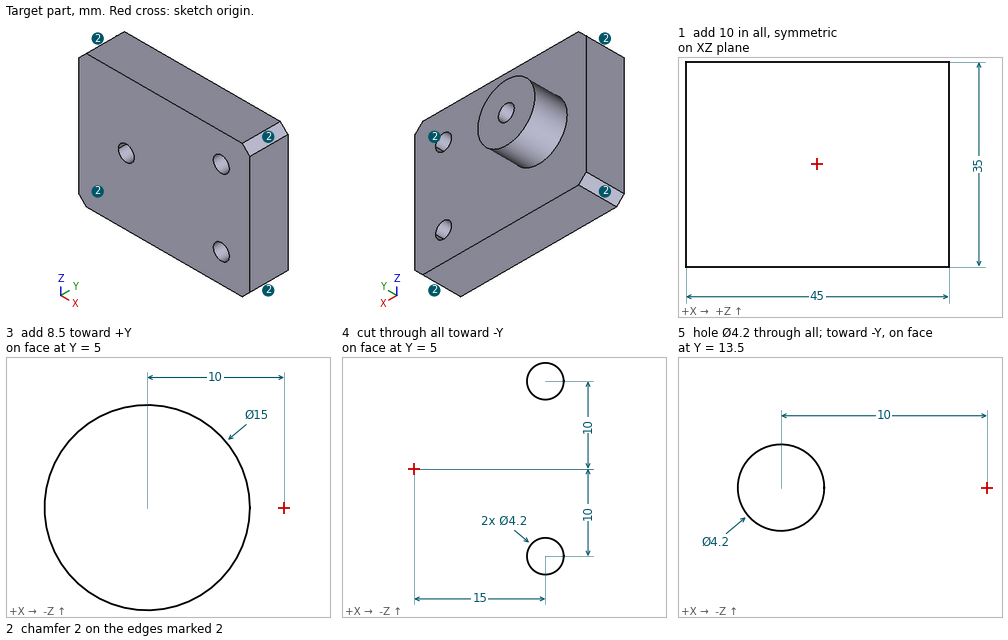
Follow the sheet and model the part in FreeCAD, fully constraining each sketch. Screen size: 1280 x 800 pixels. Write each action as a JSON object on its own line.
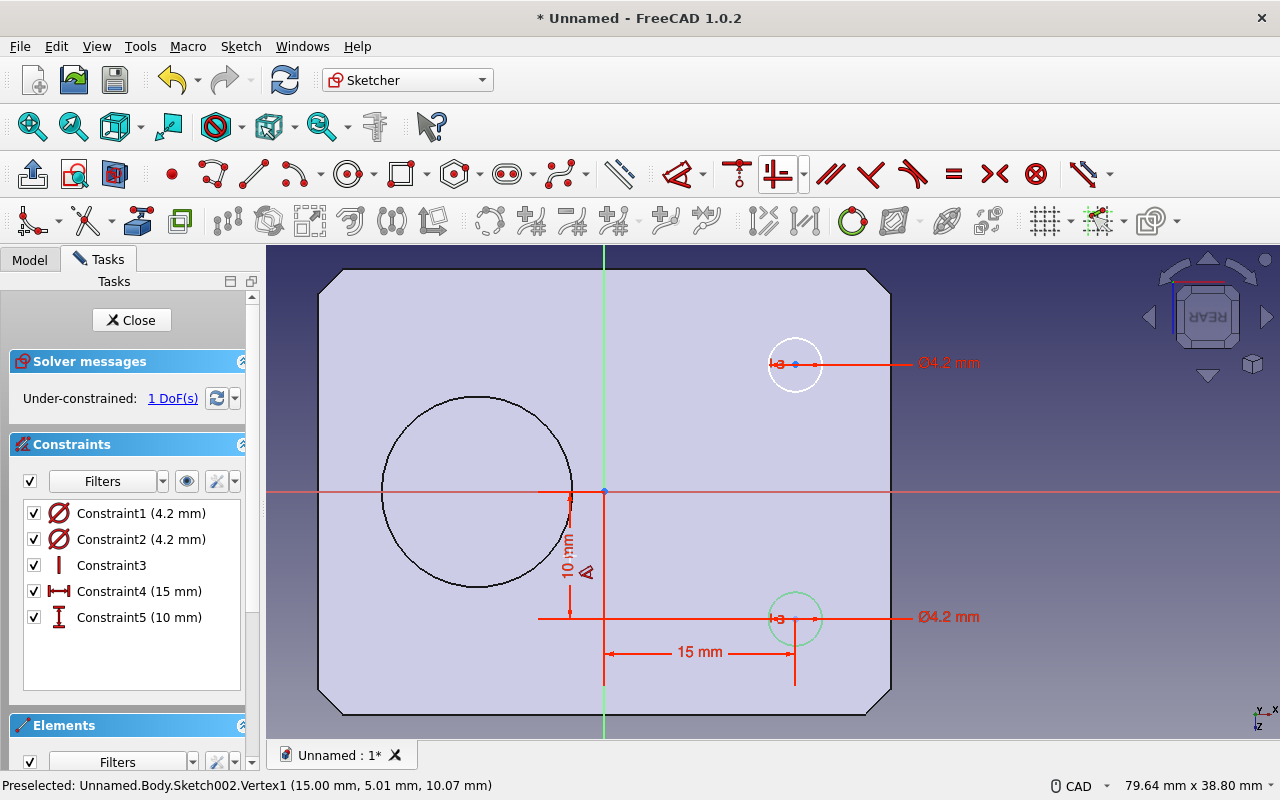
{"action": "left_click", "coordinate": [795, 365]}
{"action": "left_click", "coordinate": [570, 428]}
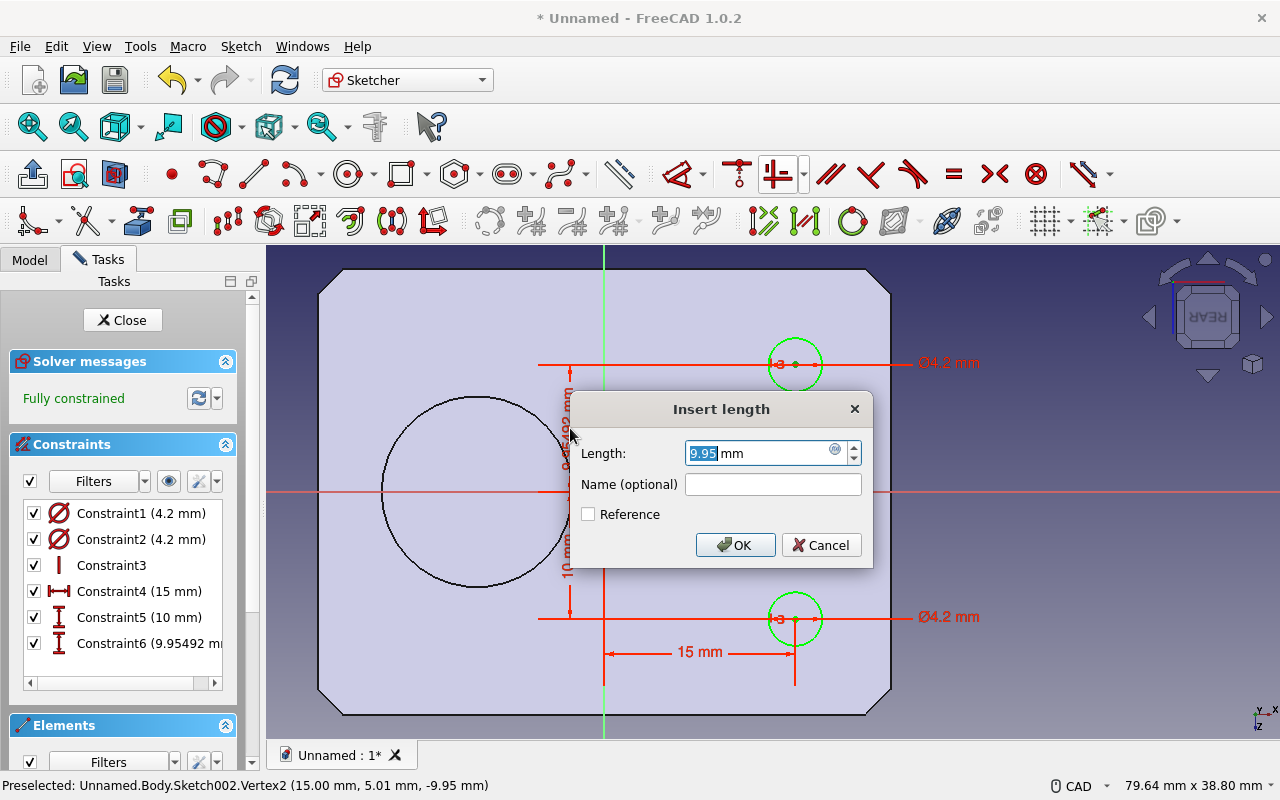
{"action": "type", "text": "10"}
{"action": "key", "text": "Return"}
{"action": "key", "text": "Escape"}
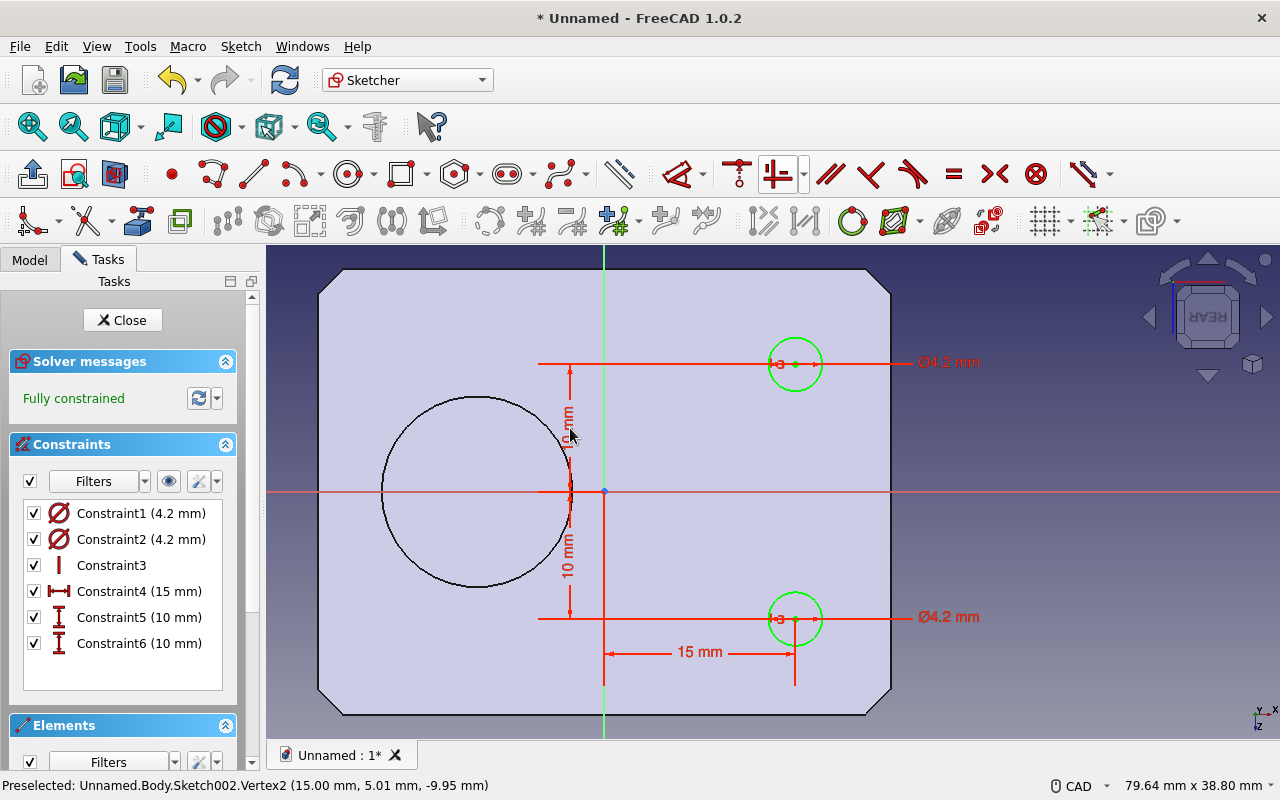
{"action": "left_click", "coordinate": [123, 320]}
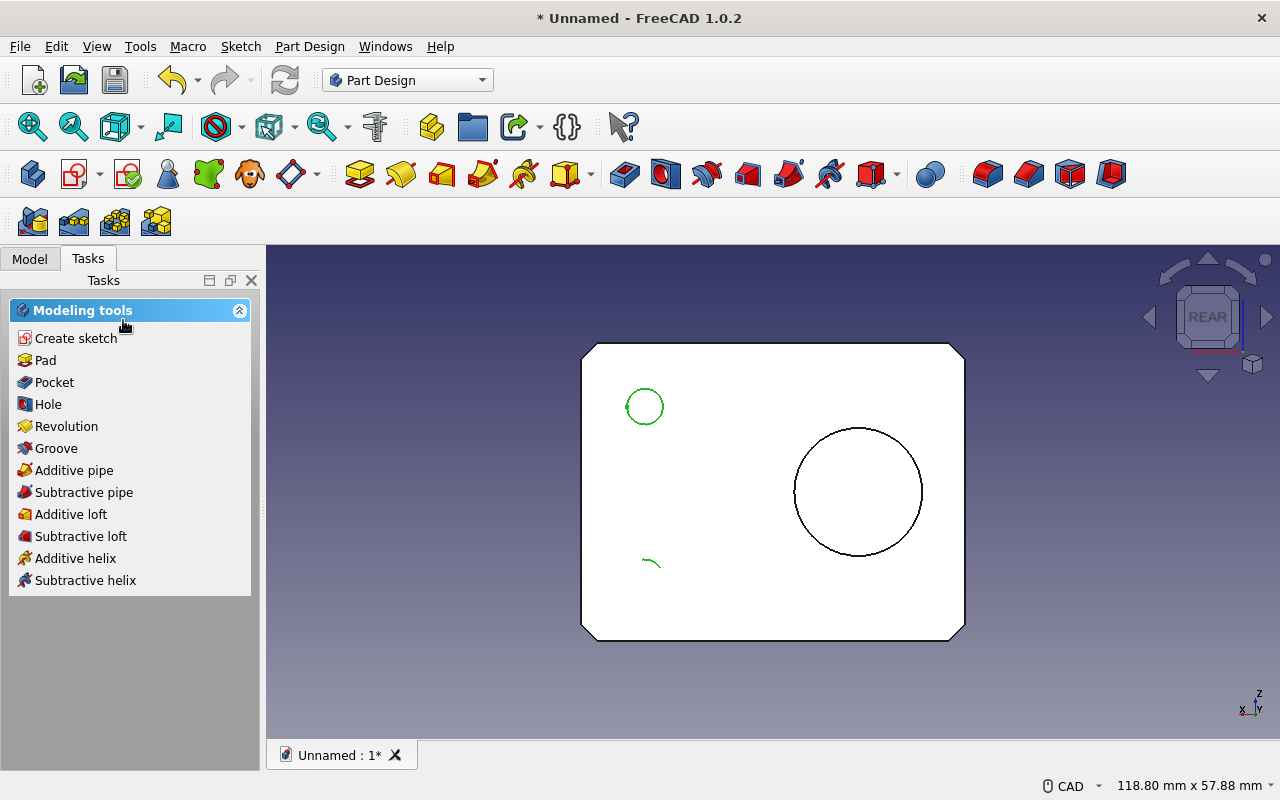
{"action": "left_click", "coordinate": [625, 174]}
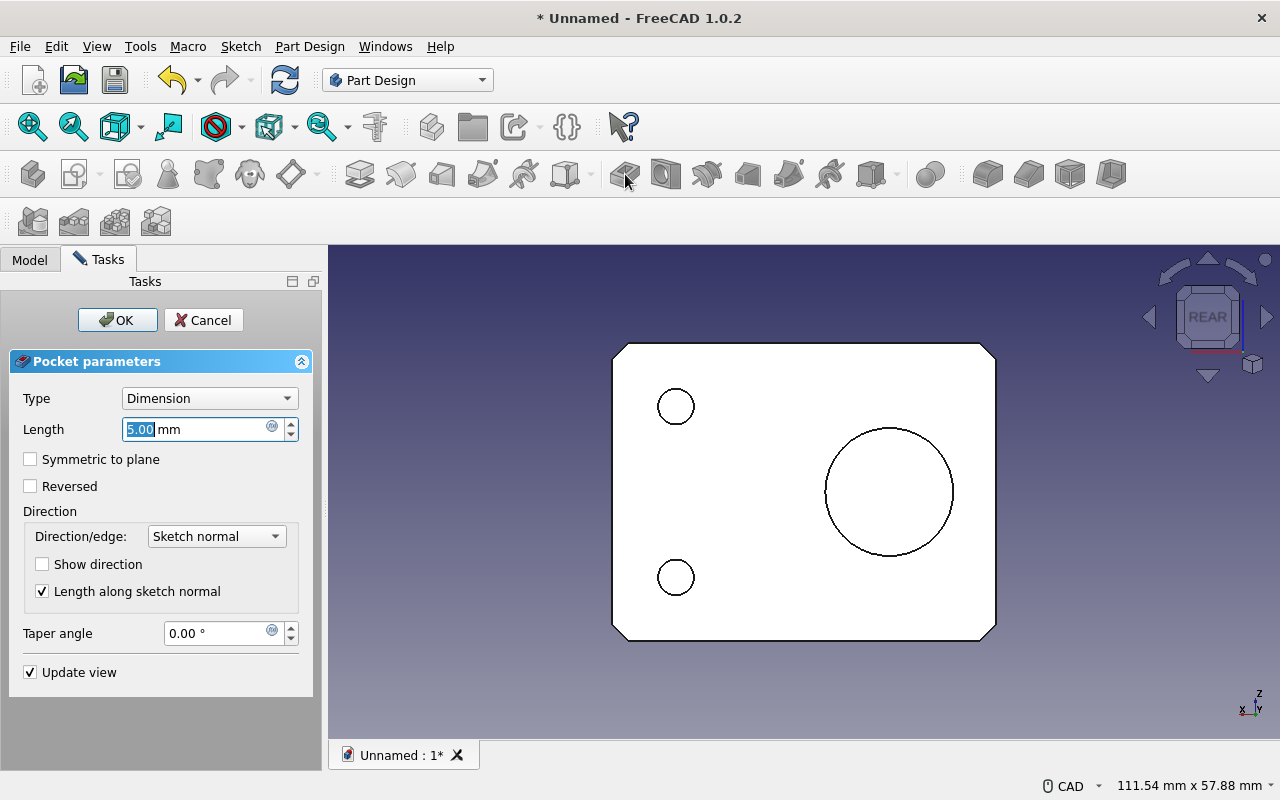
{"action": "left_click", "coordinate": [210, 398]}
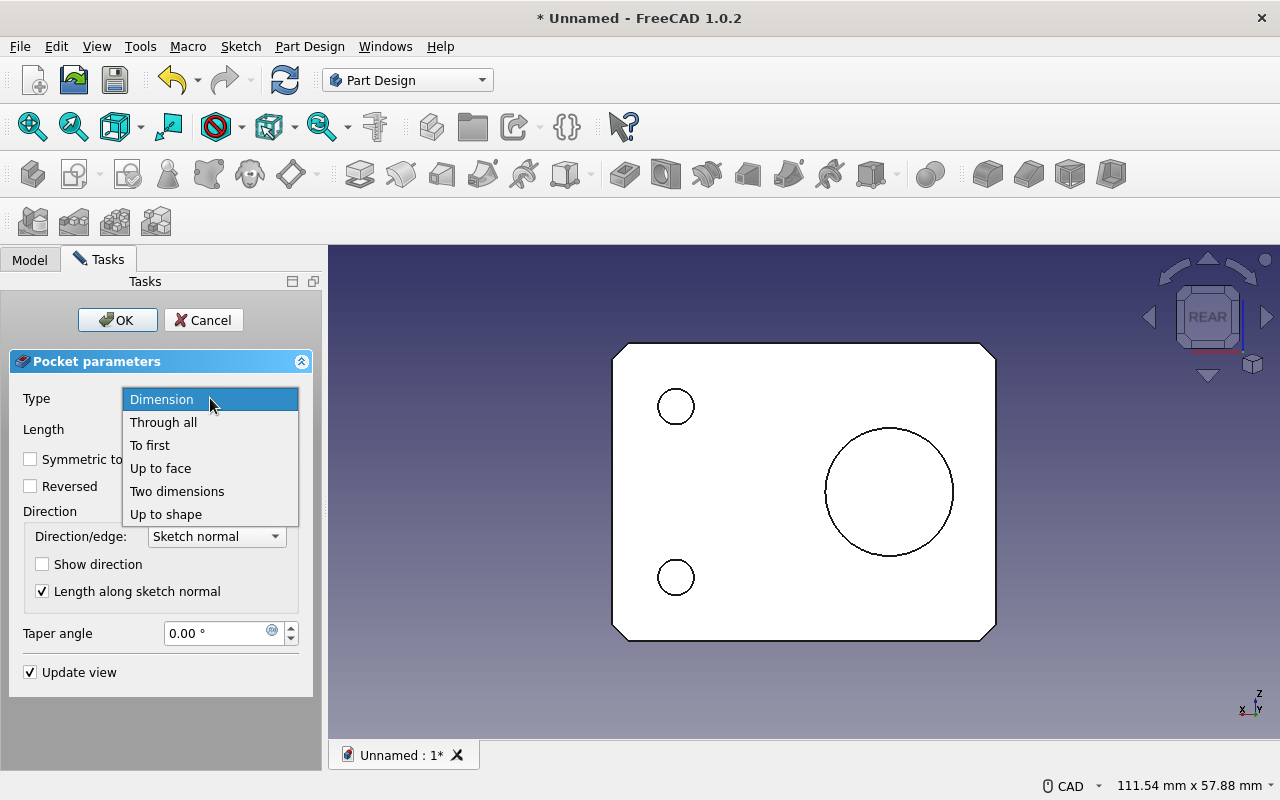
{"action": "left_click", "coordinate": [208, 422]}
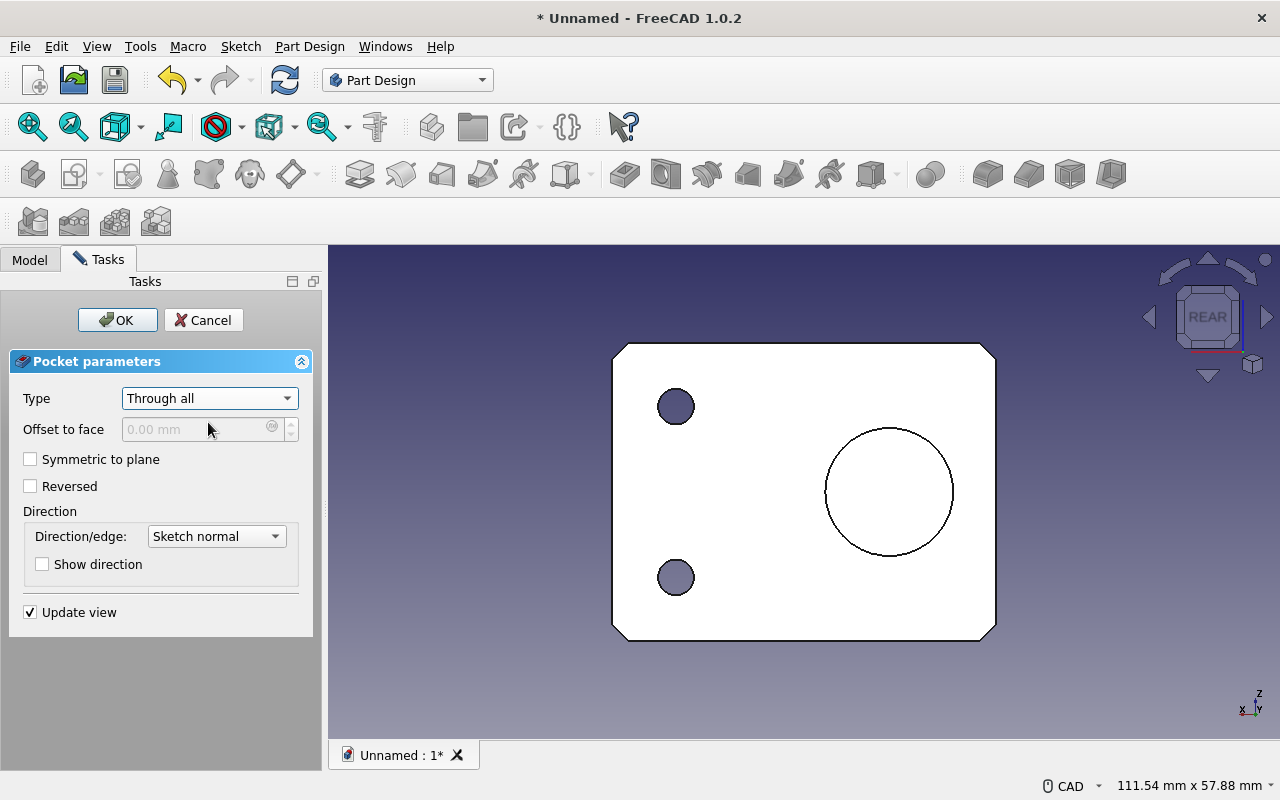
{"action": "left_click", "coordinate": [118, 320]}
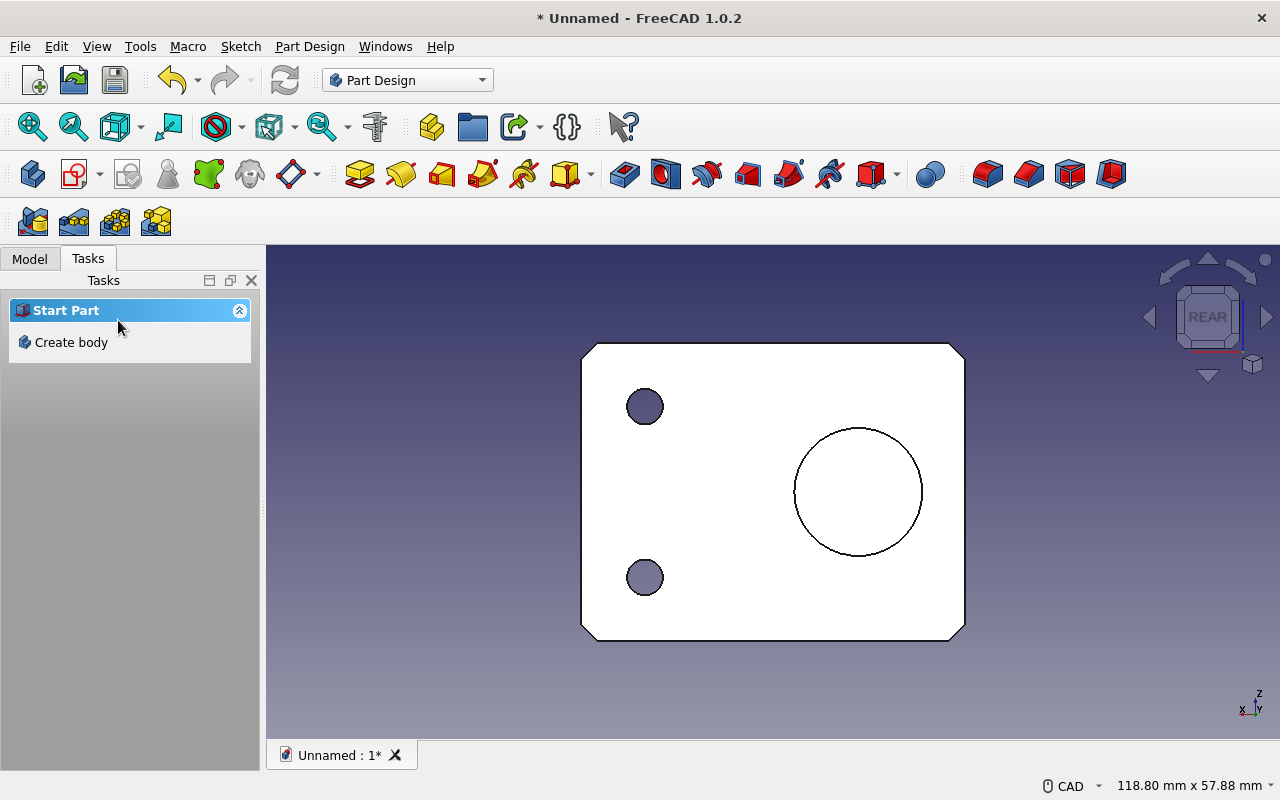
{"action": "left_click", "coordinate": [858, 491]}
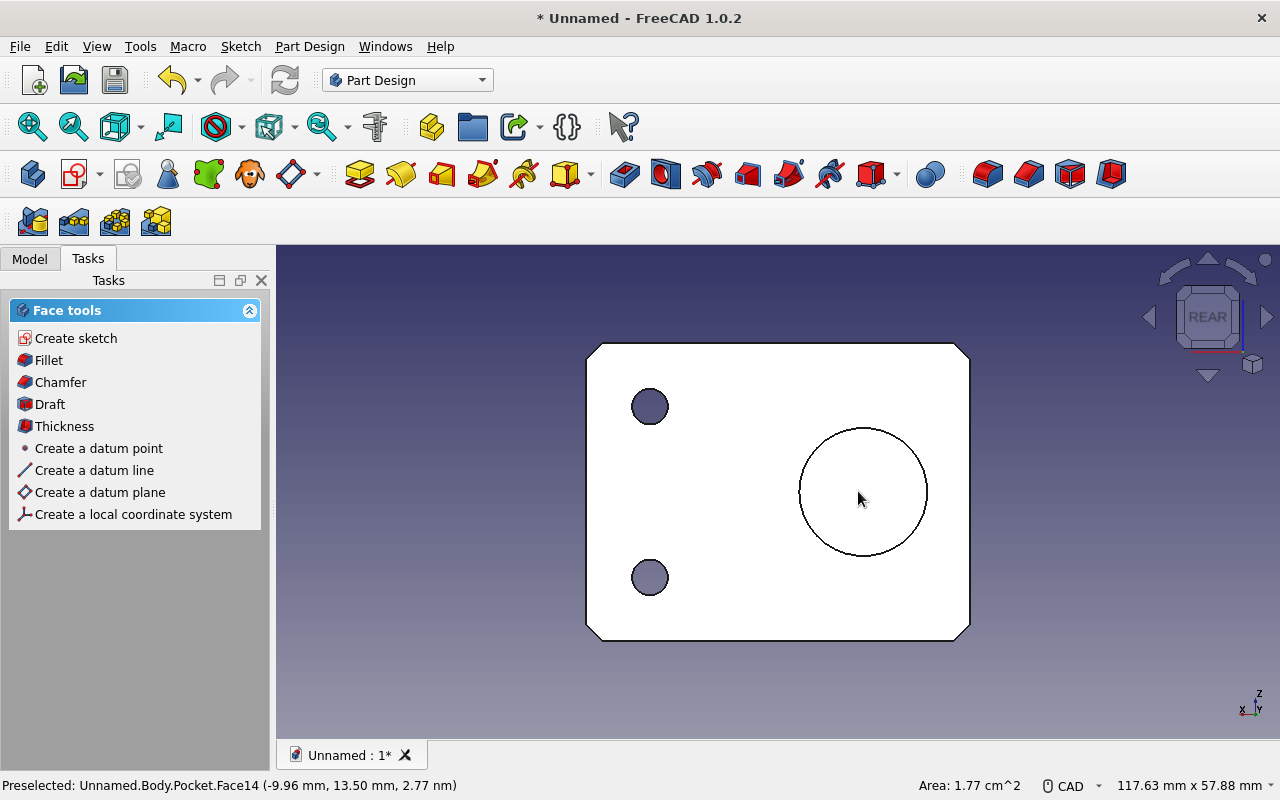
{"action": "left_click", "coordinate": [74, 174]}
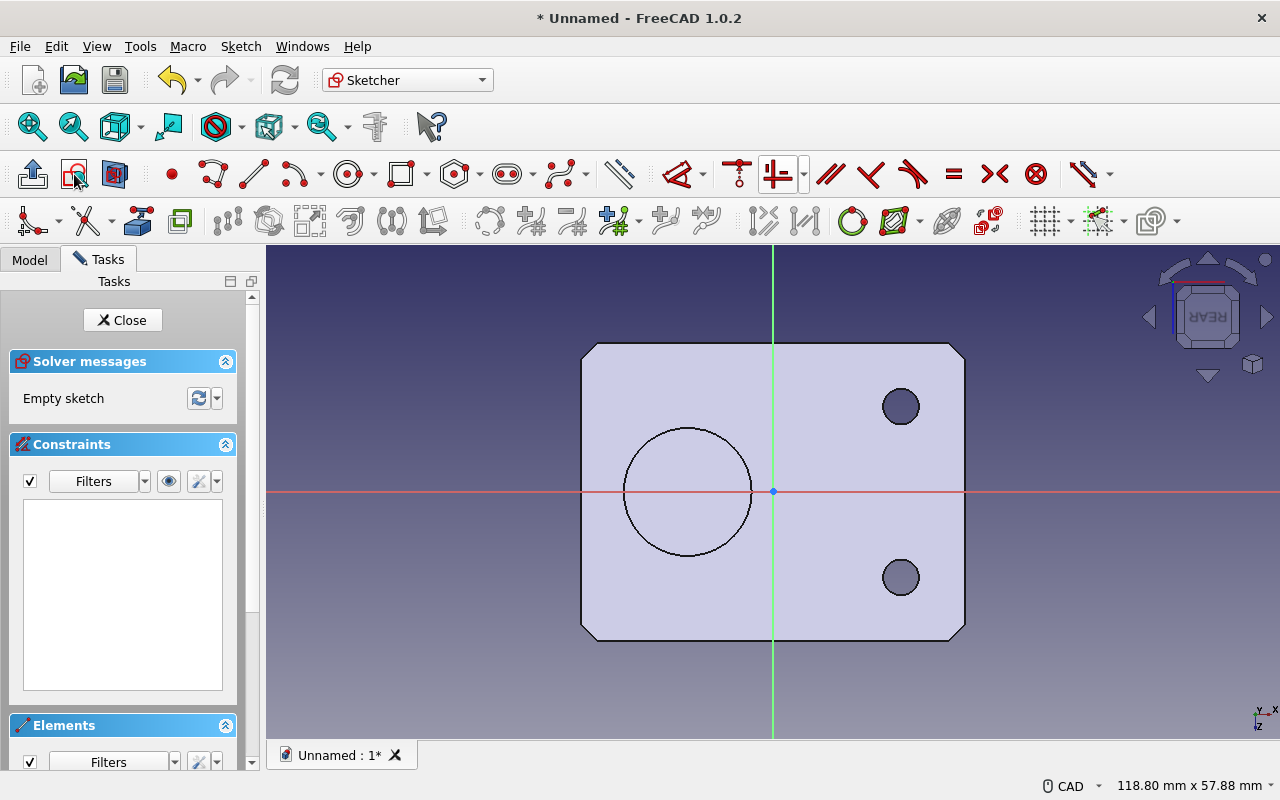
{"action": "scroll", "coordinate": [686, 492], "scroll_direction": "up", "scroll_amount": 11}